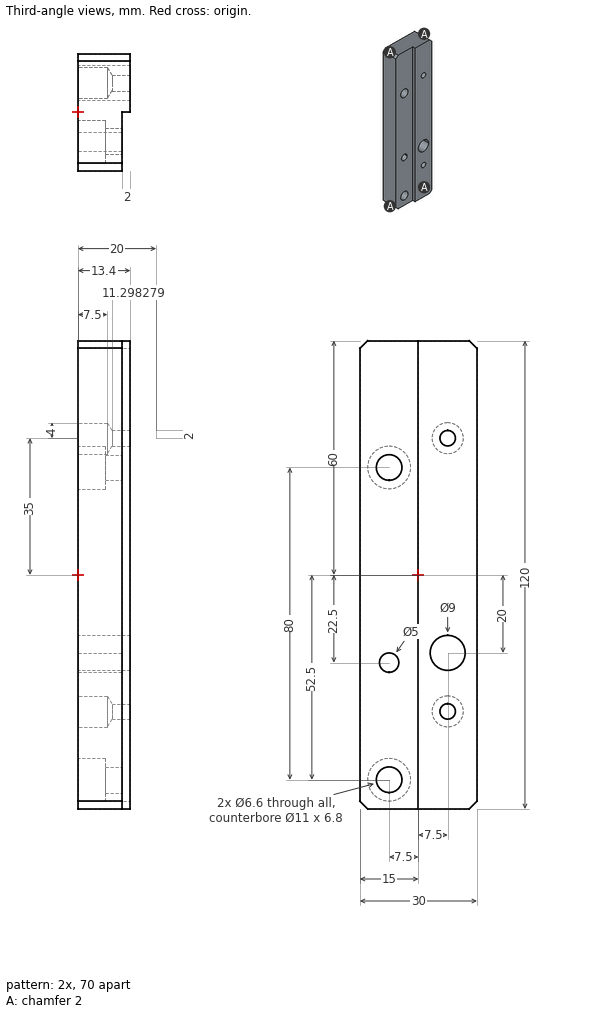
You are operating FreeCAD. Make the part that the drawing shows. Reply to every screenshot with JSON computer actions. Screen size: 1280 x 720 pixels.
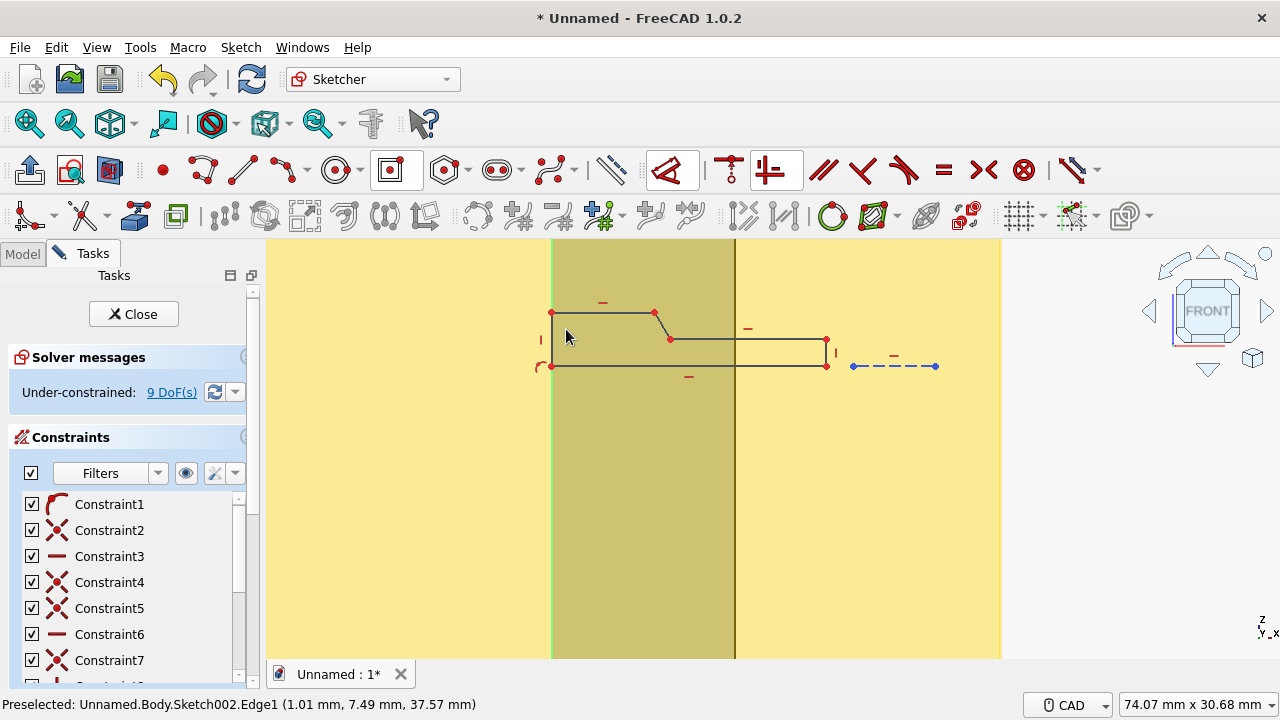
{"action": "left_click", "coordinate": [552, 350]}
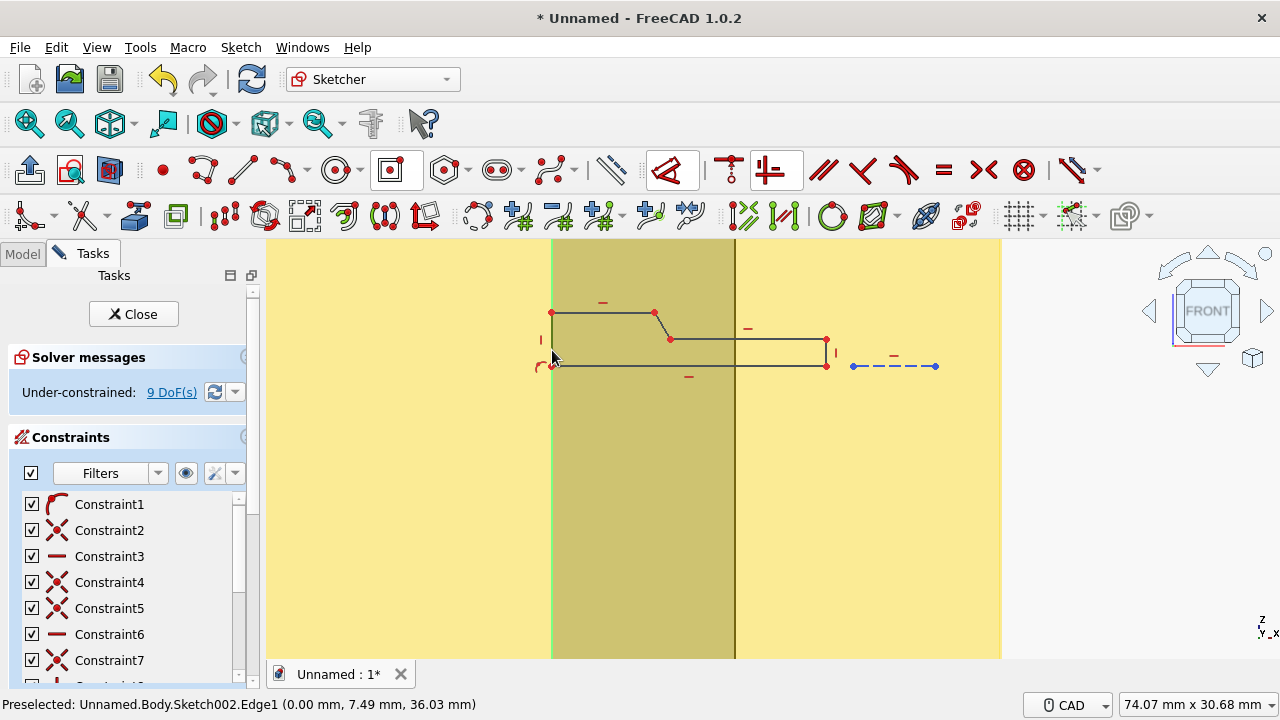
{"action": "left_click", "coordinate": [694, 170]}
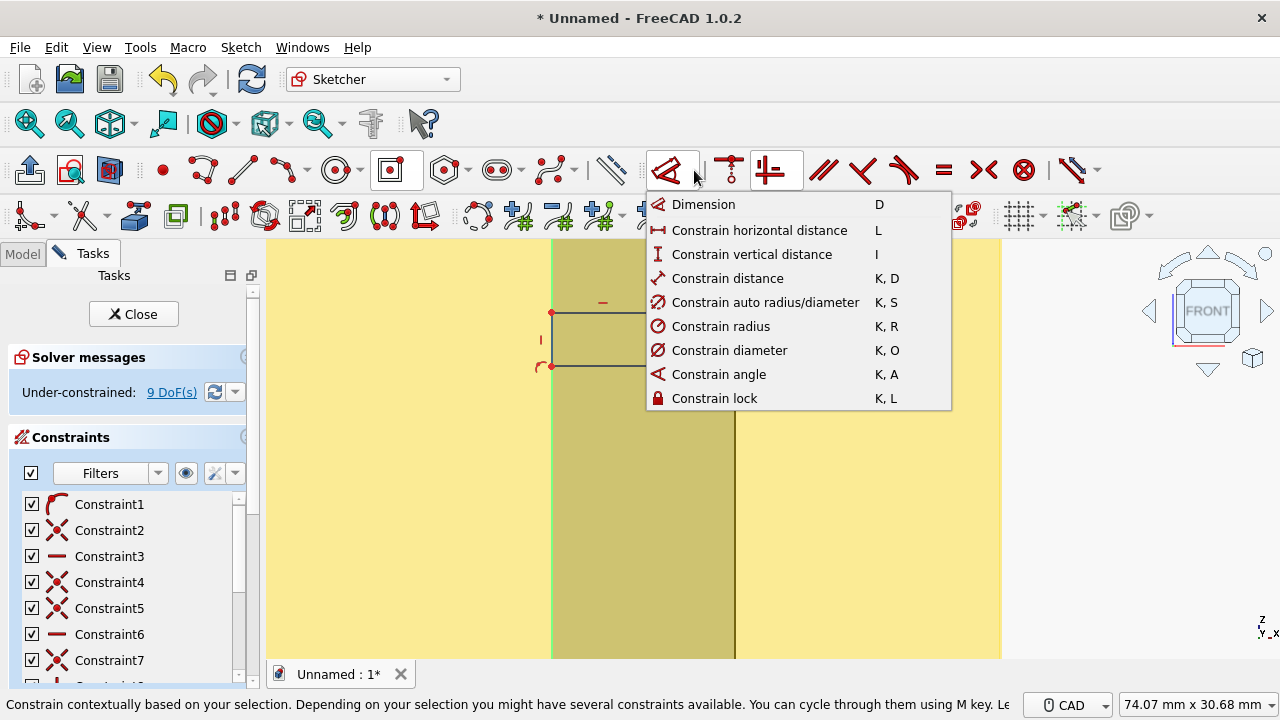
{"action": "left_click", "coordinate": [799, 254]}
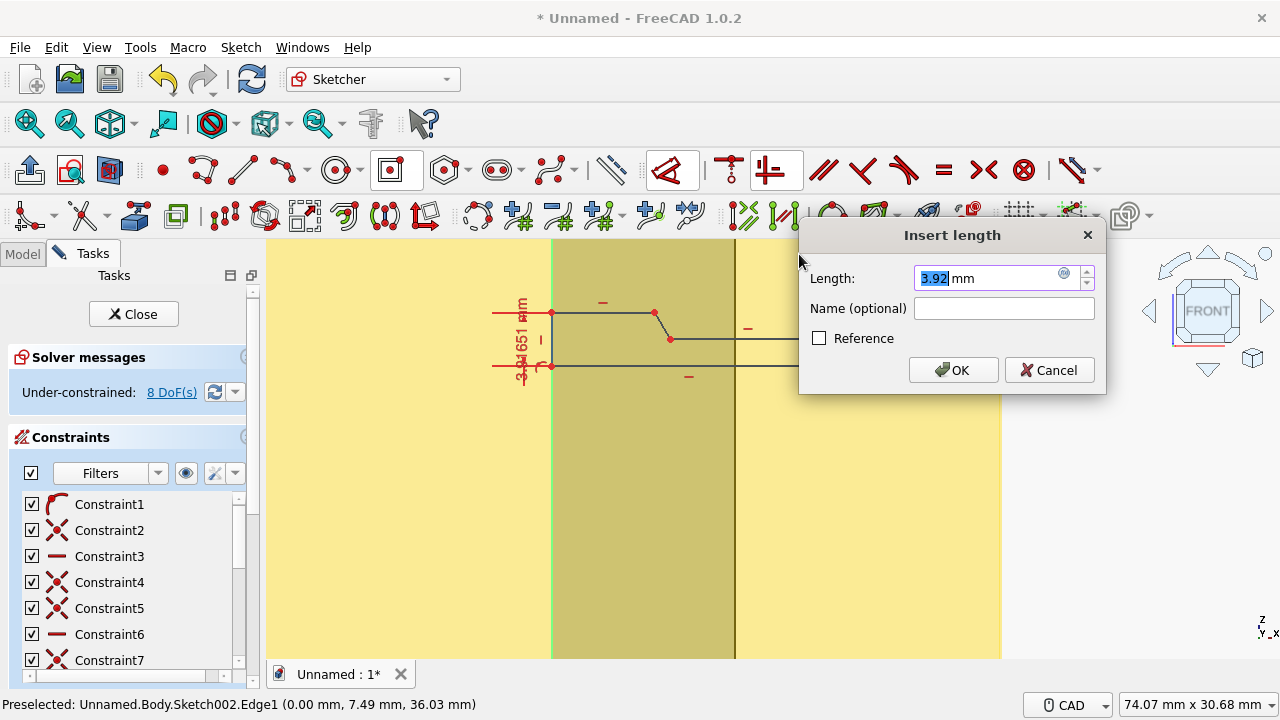
{"action": "type", "text": "4"}
{"action": "key", "text": "Return"}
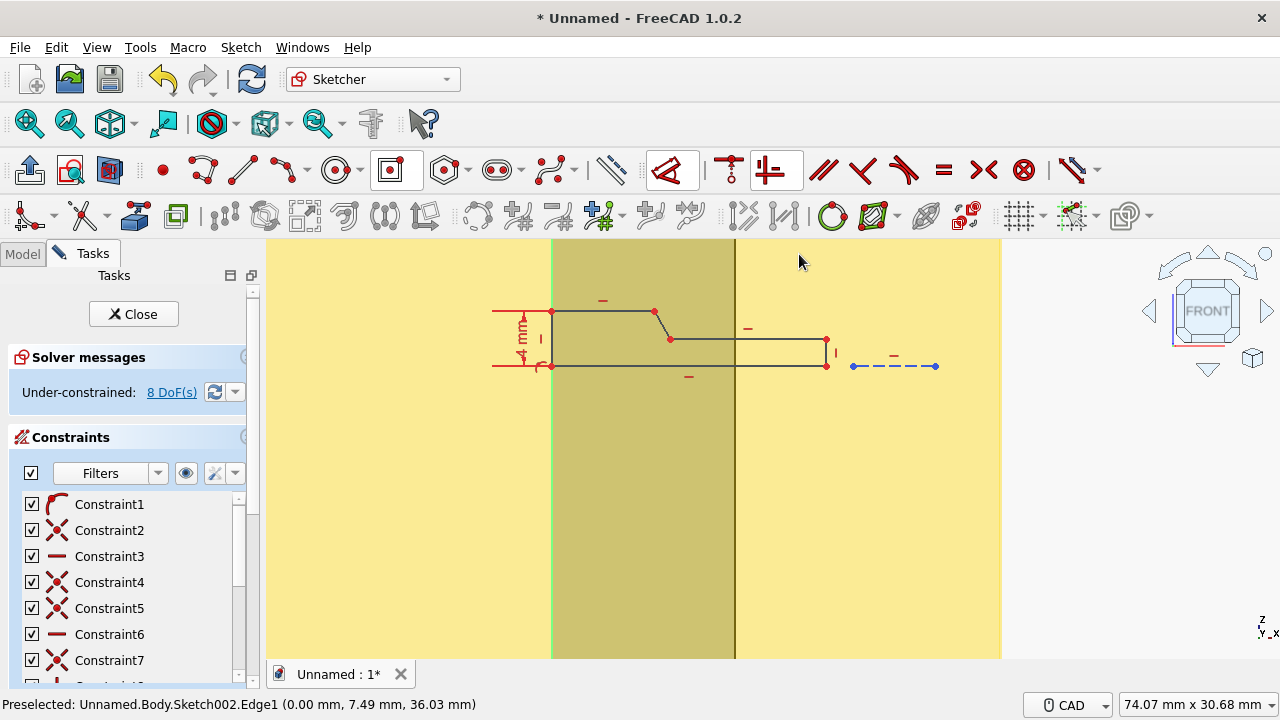
{"action": "scroll", "coordinate": [826, 350], "scroll_direction": "up", "scroll_amount": 2}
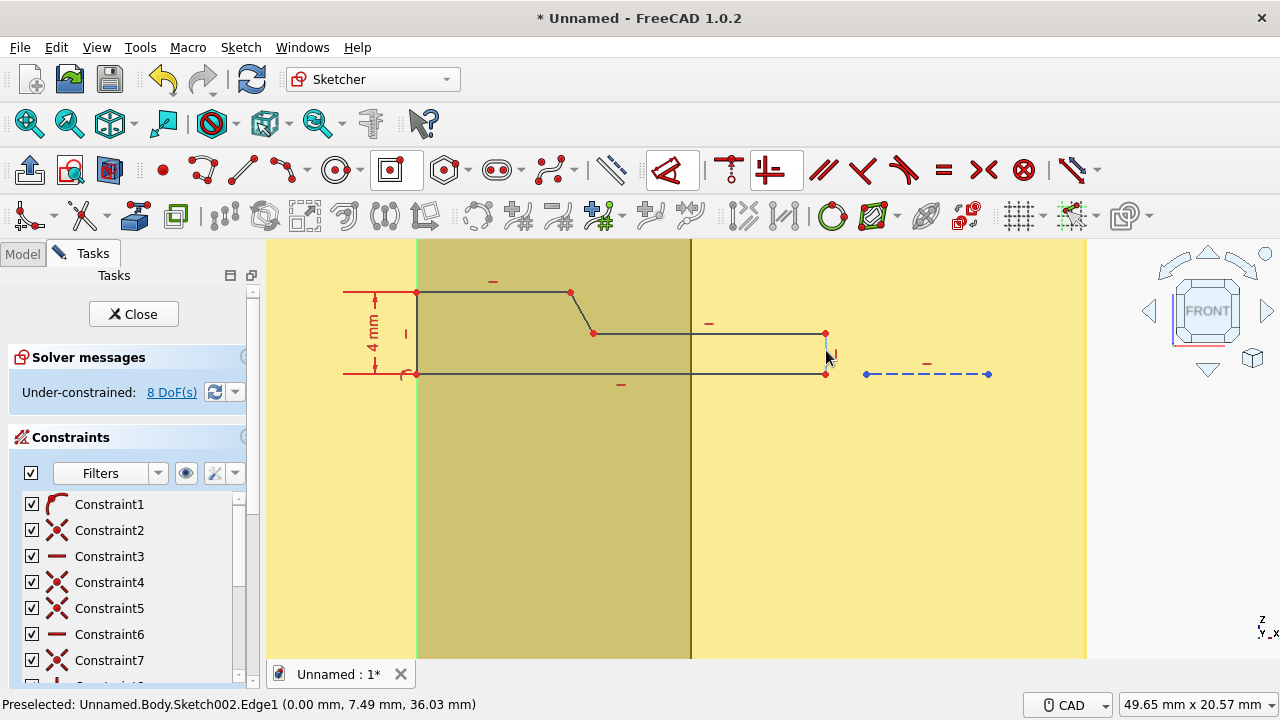
{"action": "left_click", "coordinate": [826, 350]}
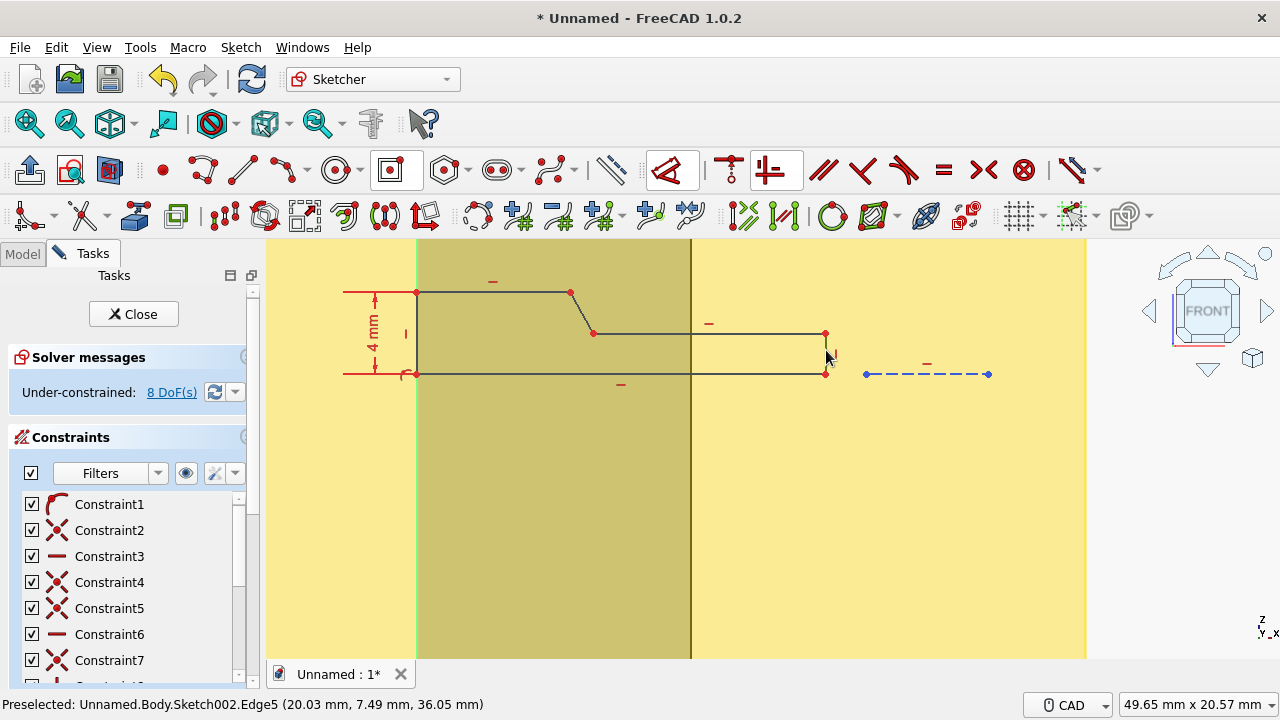
{"action": "left_click", "coordinate": [694, 170]}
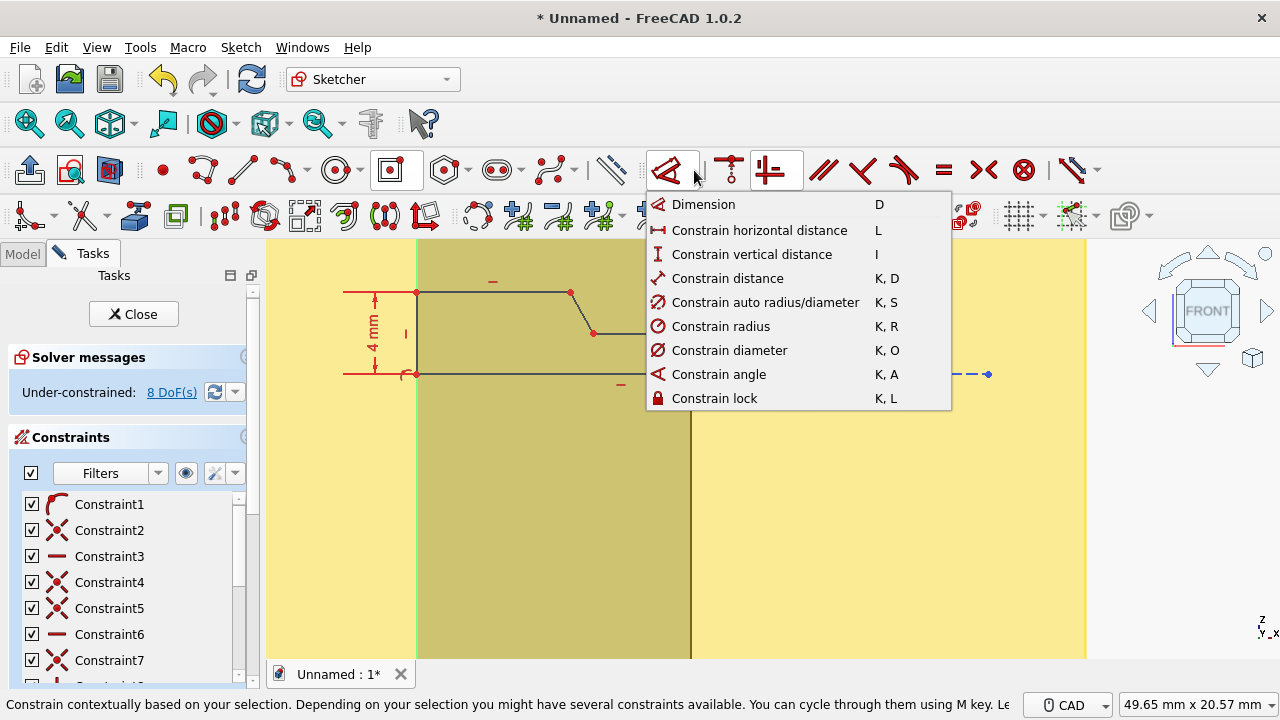
{"action": "left_click", "coordinate": [799, 254]}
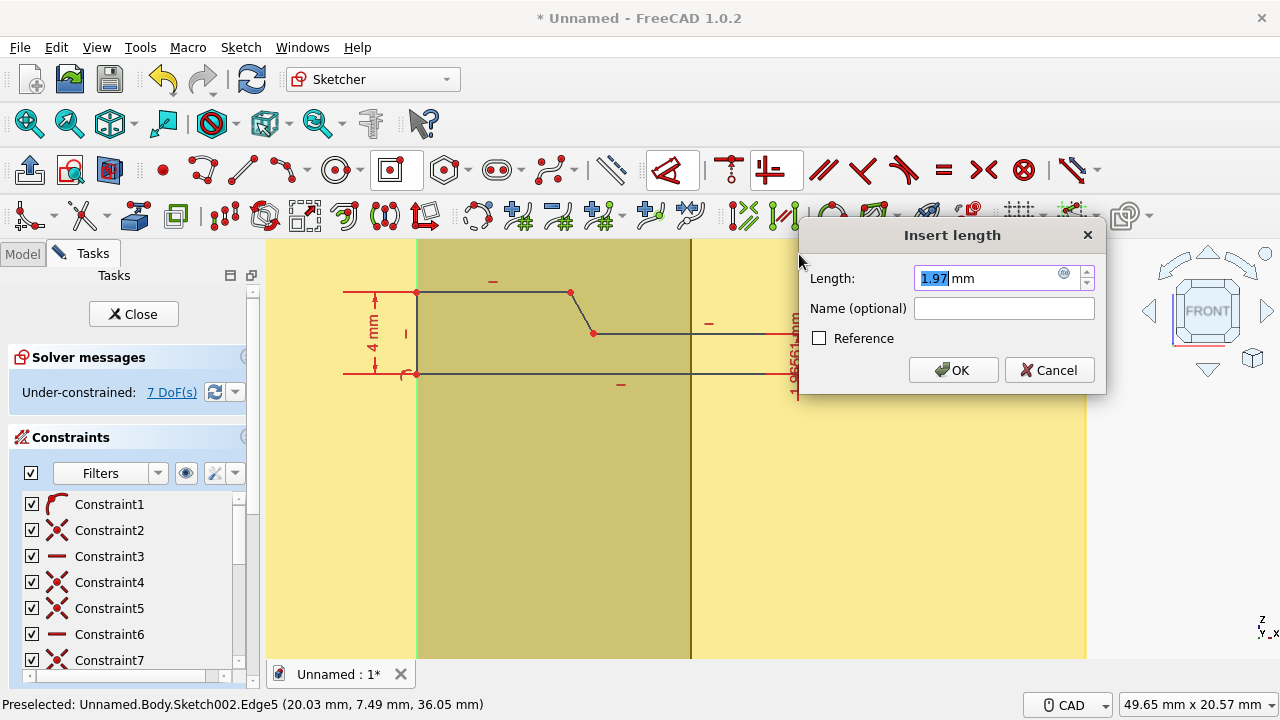
{"action": "type", "text": "2"}
{"action": "key", "text": "Return"}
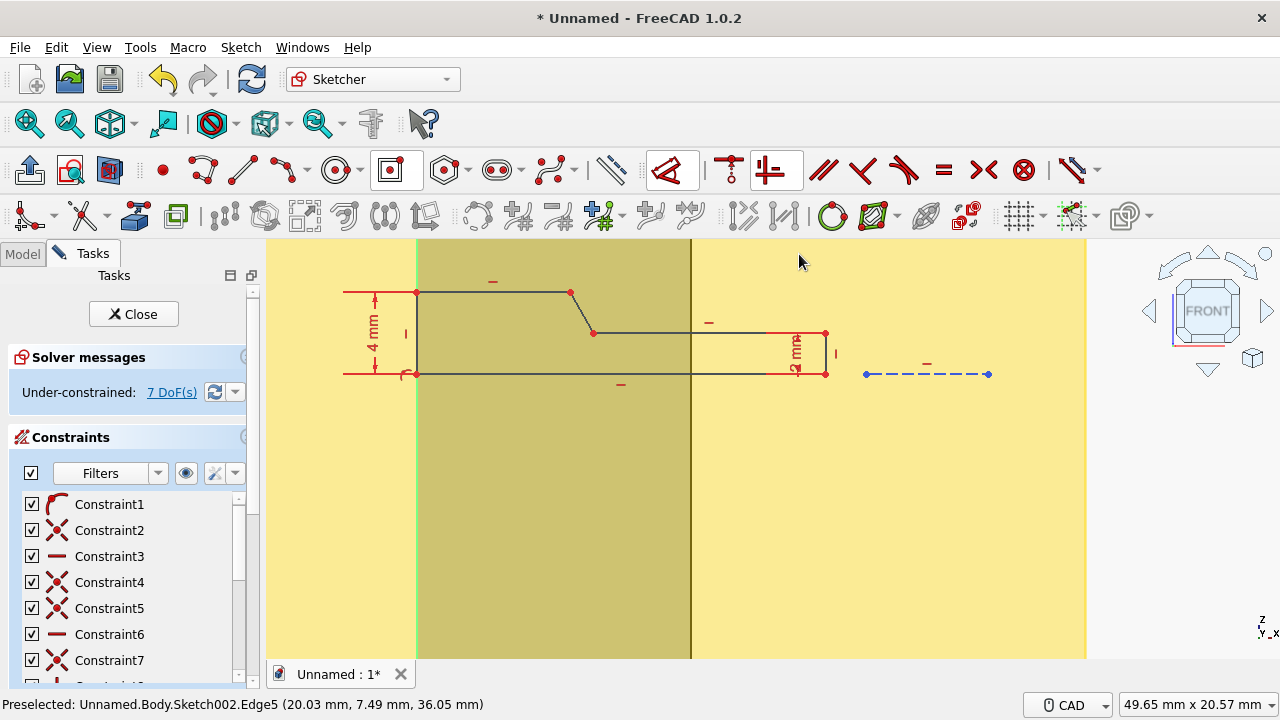
{"action": "left_click", "coordinate": [703, 374]}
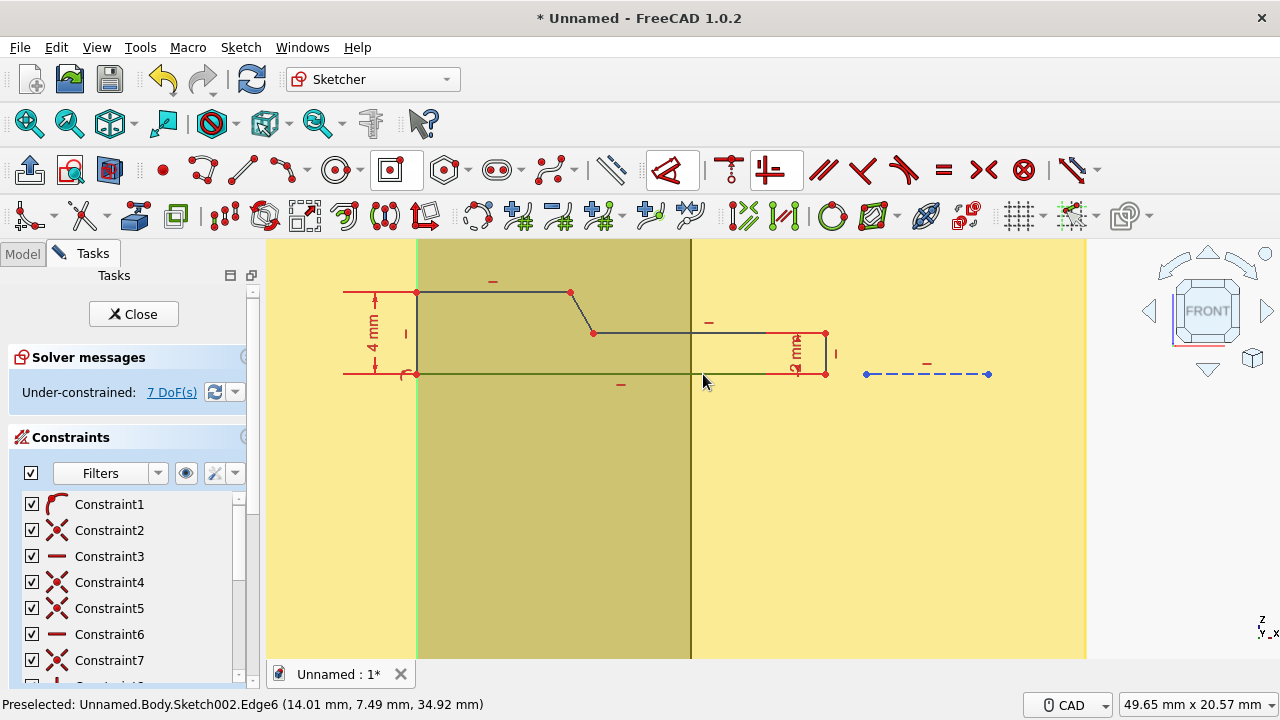
{"action": "key", "text": "l"}